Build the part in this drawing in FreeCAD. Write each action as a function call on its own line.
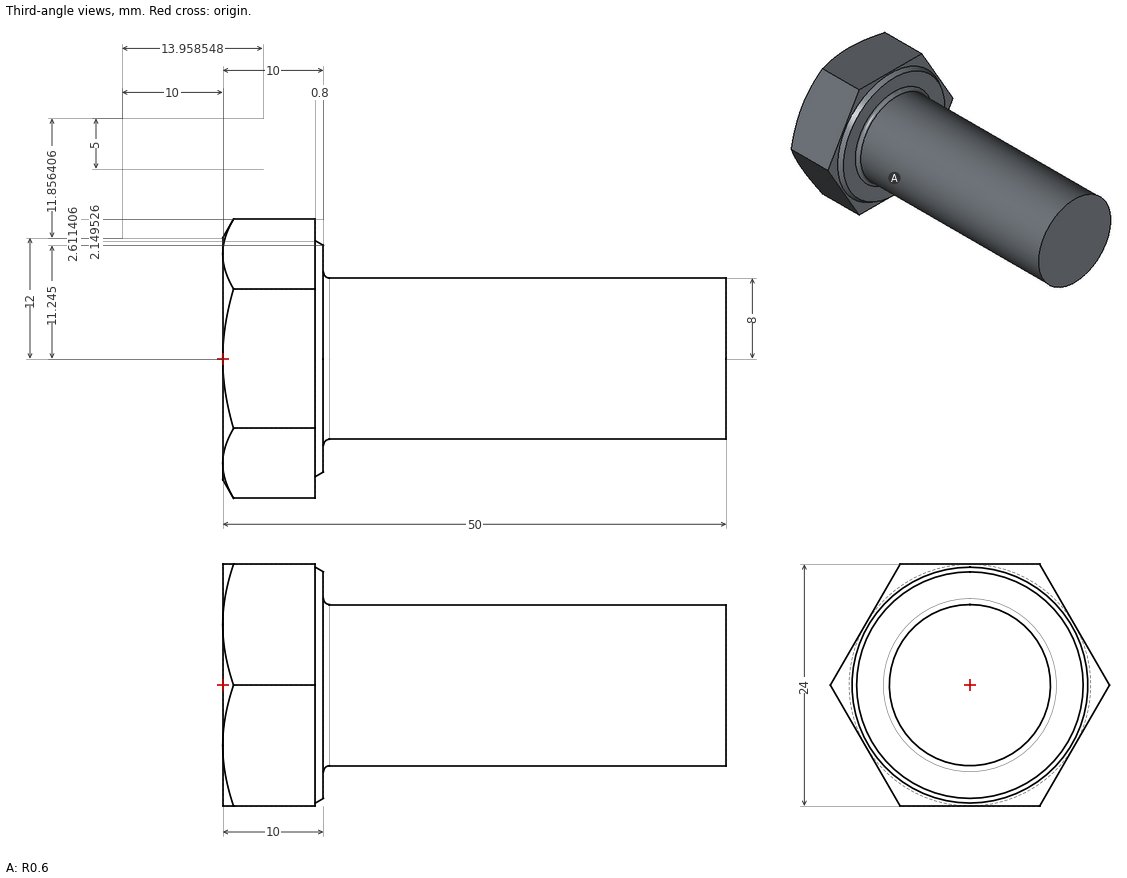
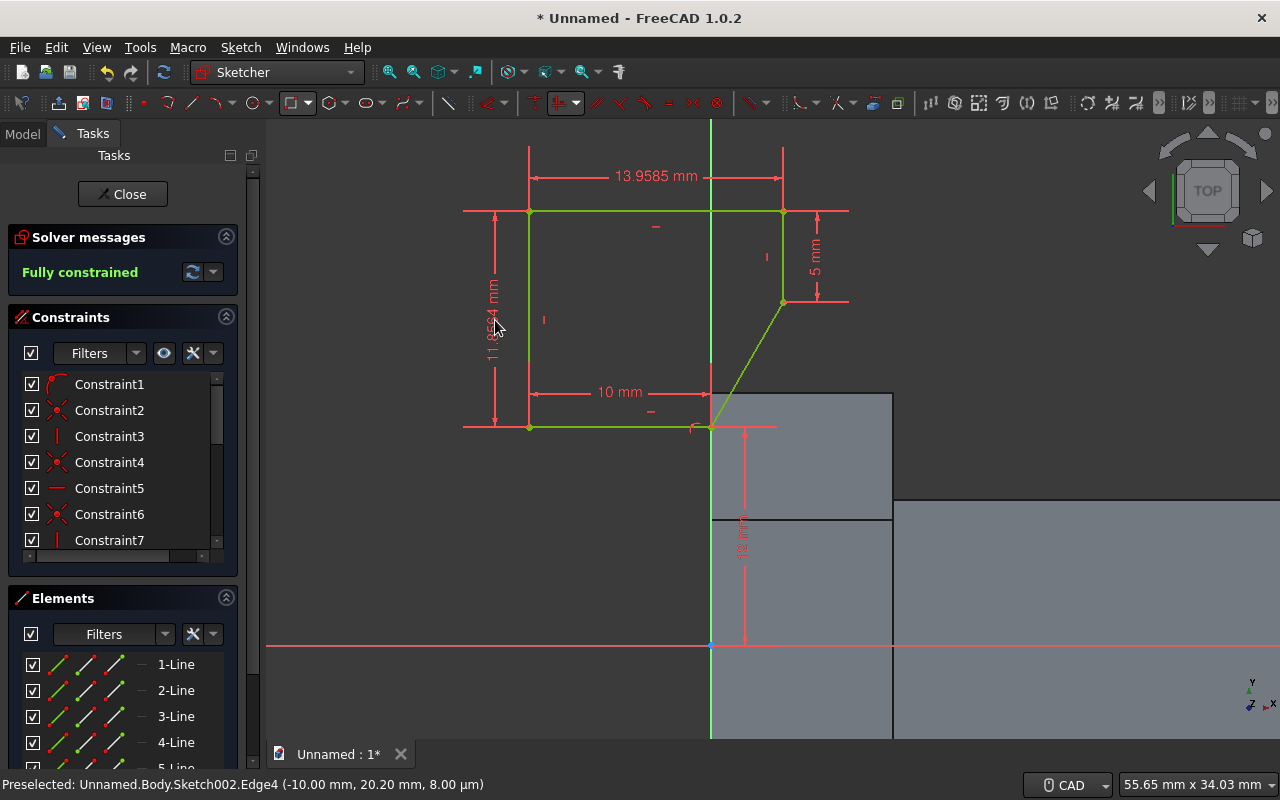
click(123, 194)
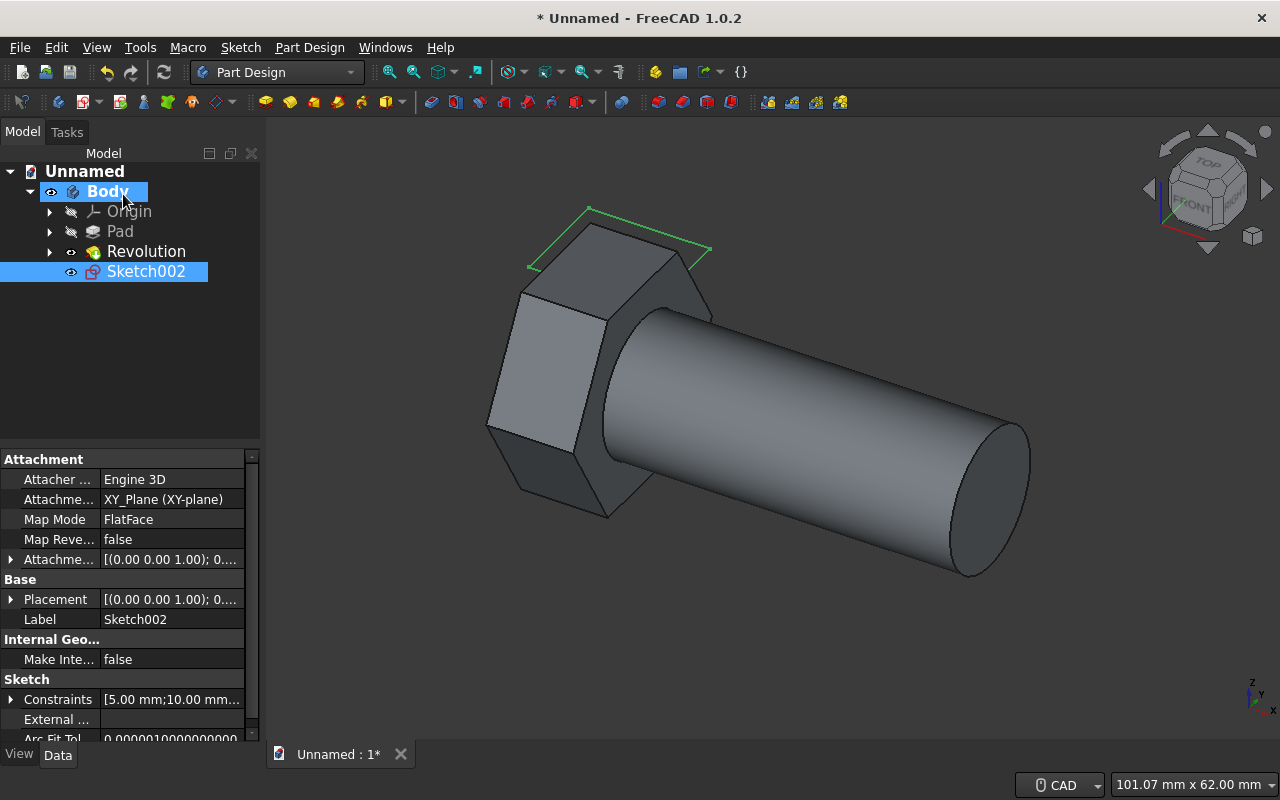
click(480, 102)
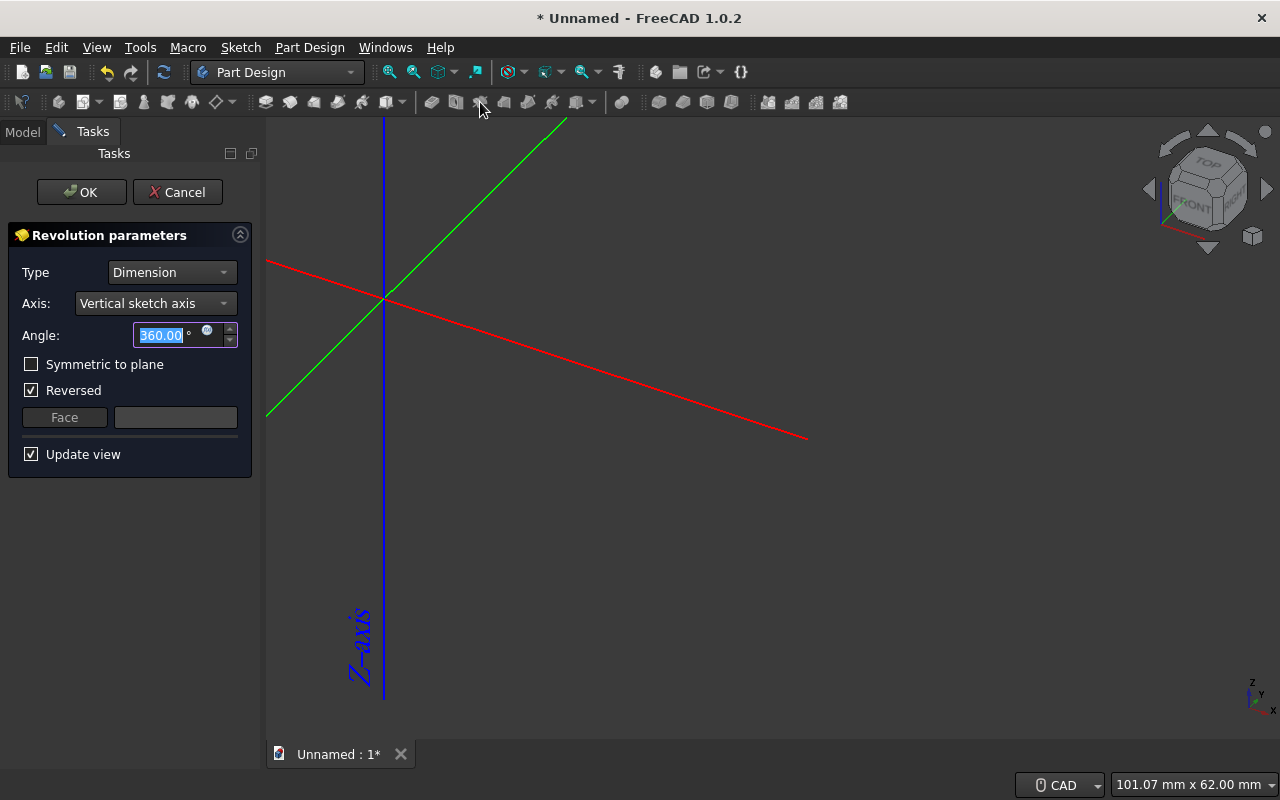
click(156, 304)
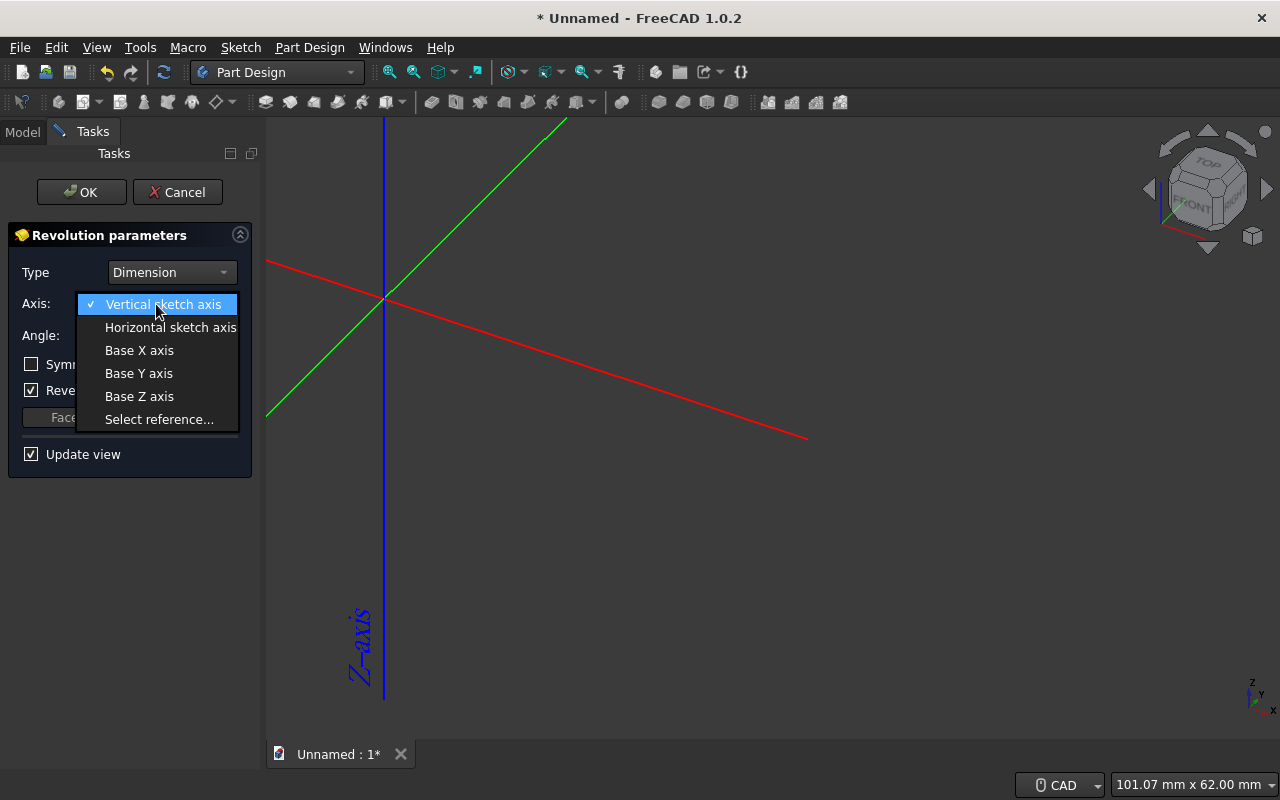
click(156, 328)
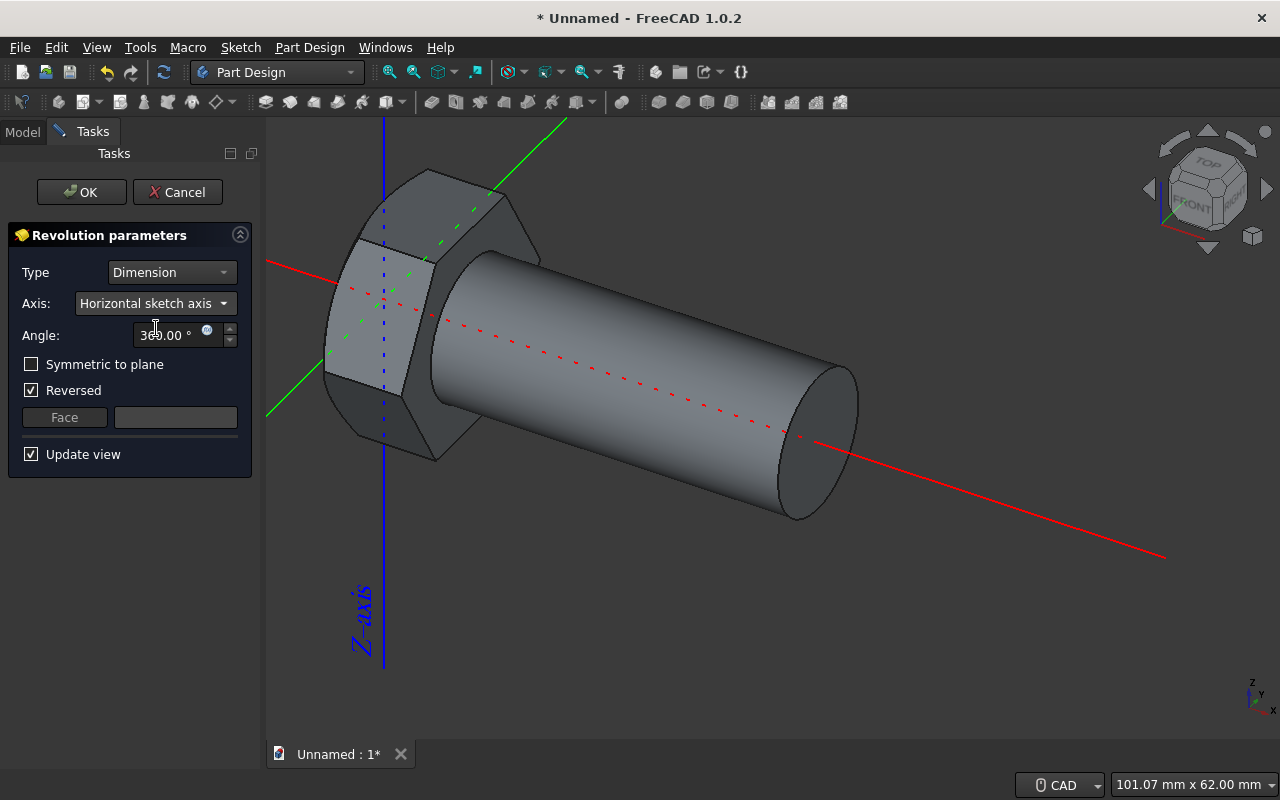
click(82, 192)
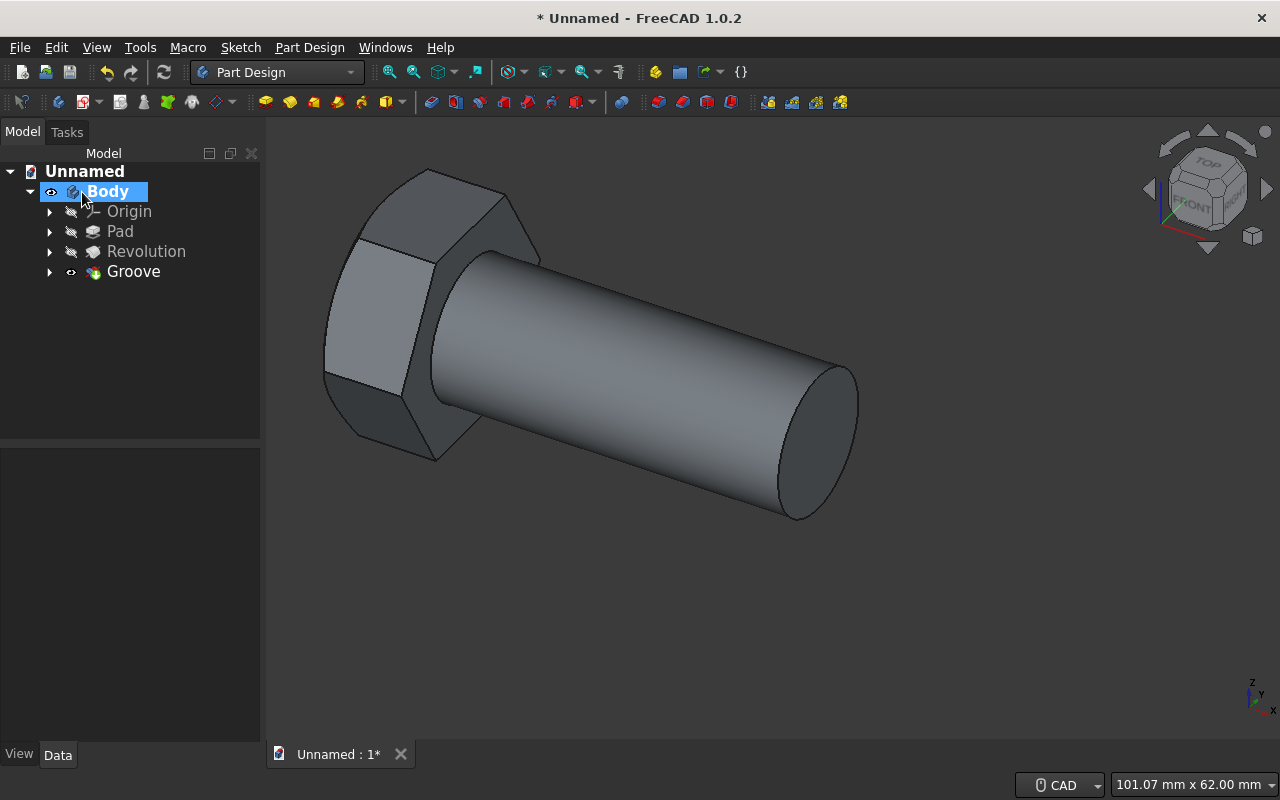
click(84, 102)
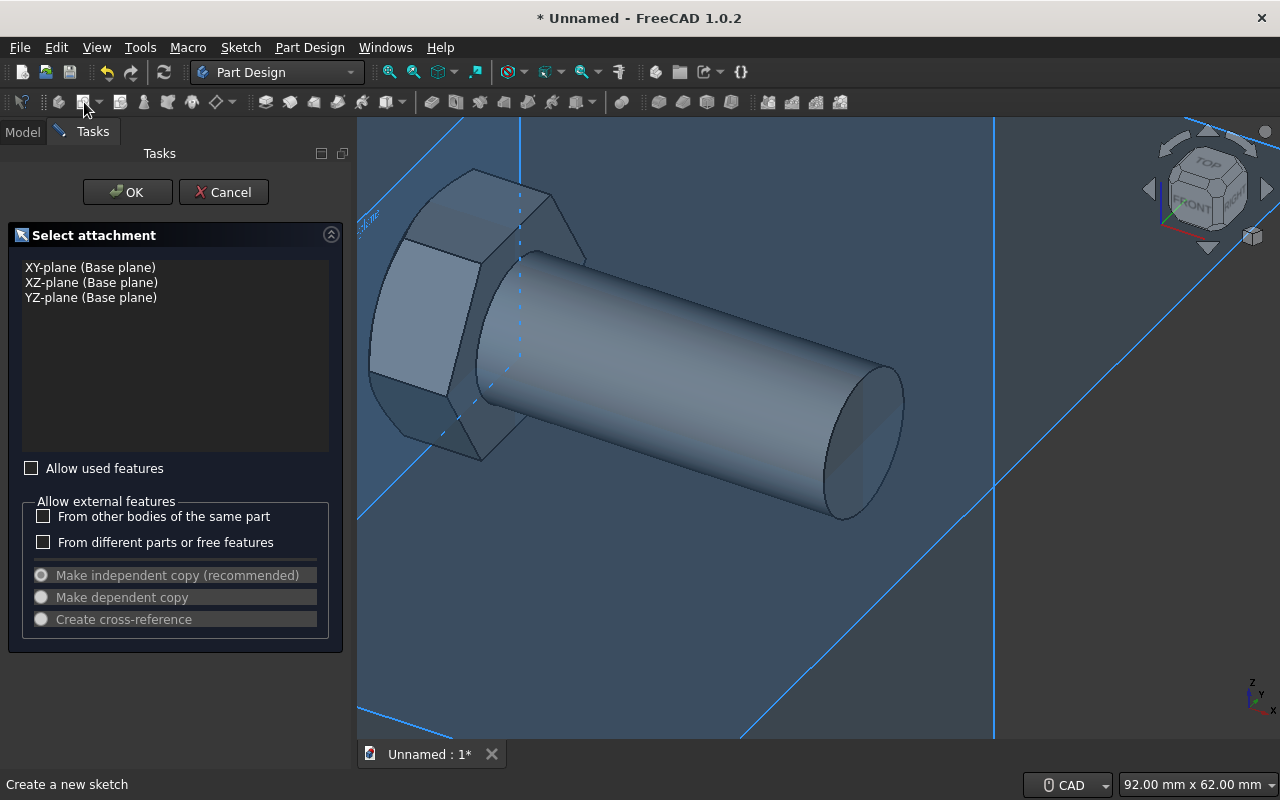
click(82, 268)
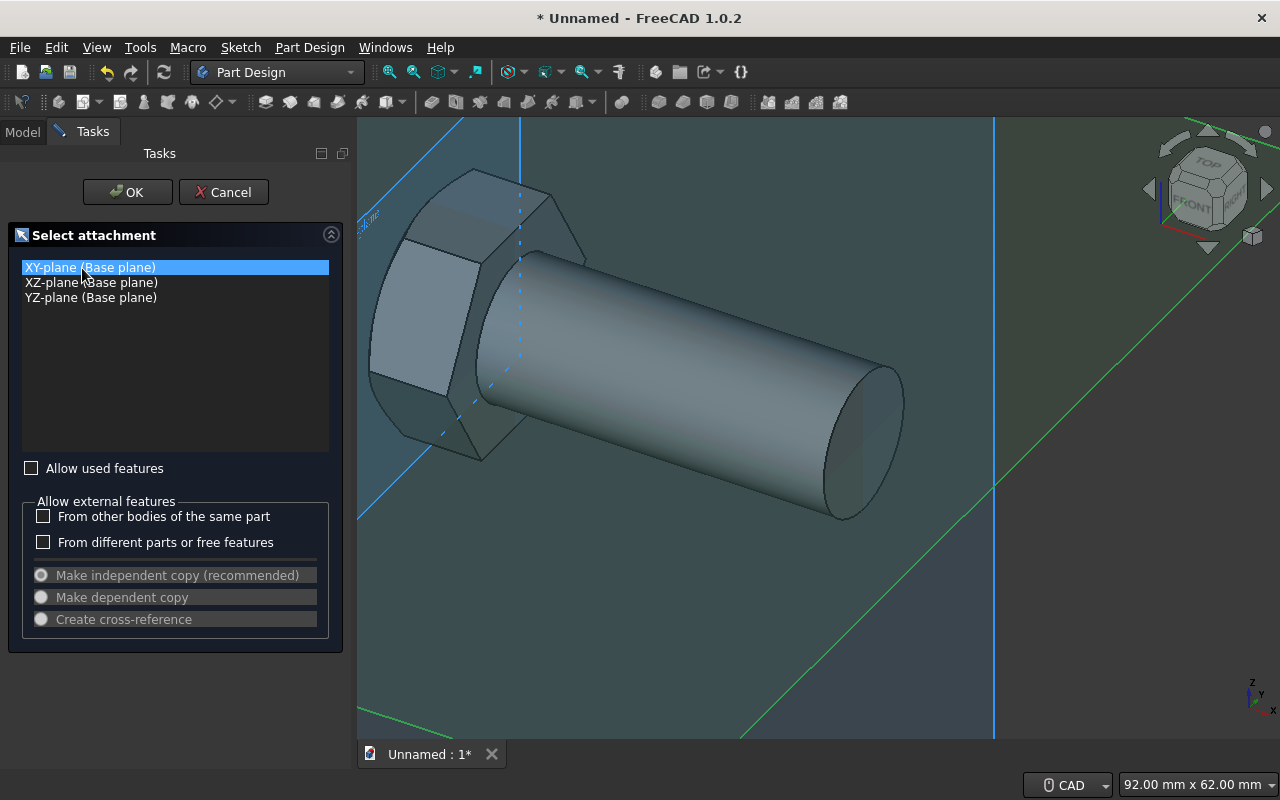
click(128, 192)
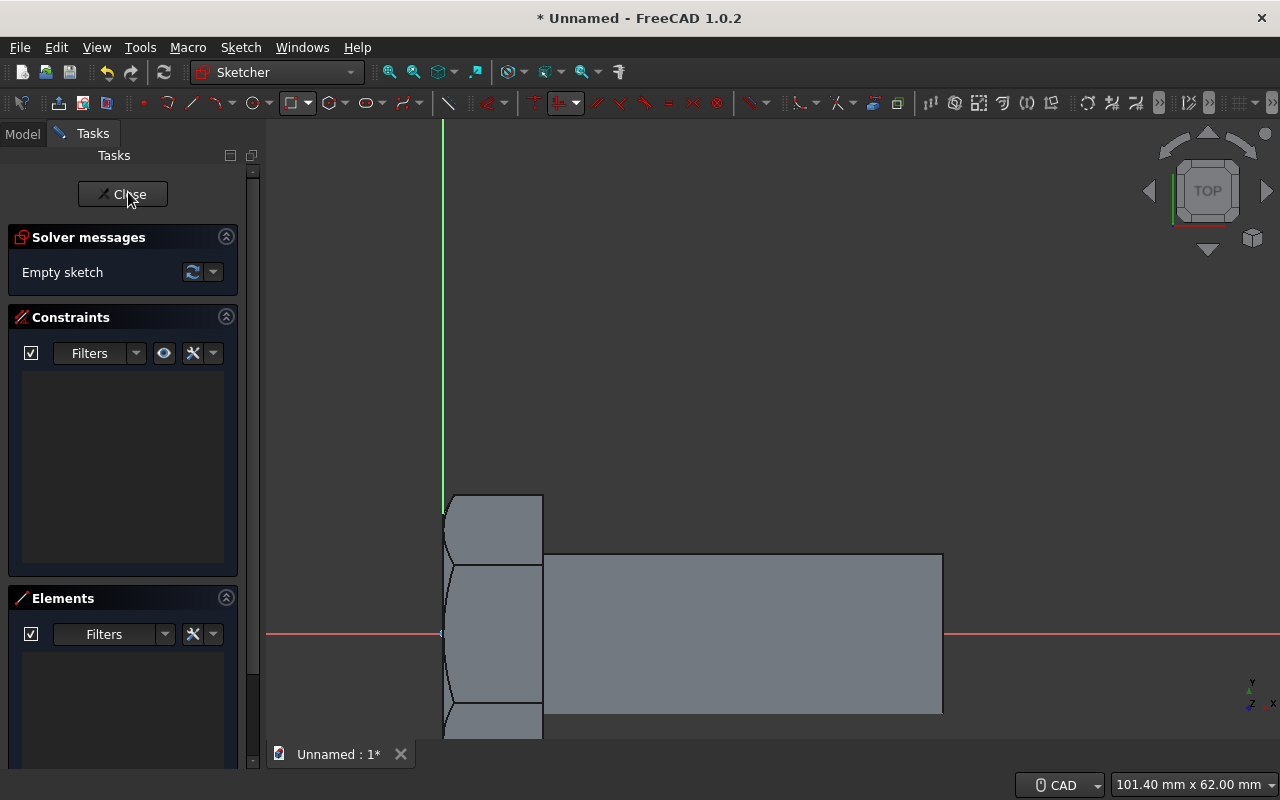
click(108, 104)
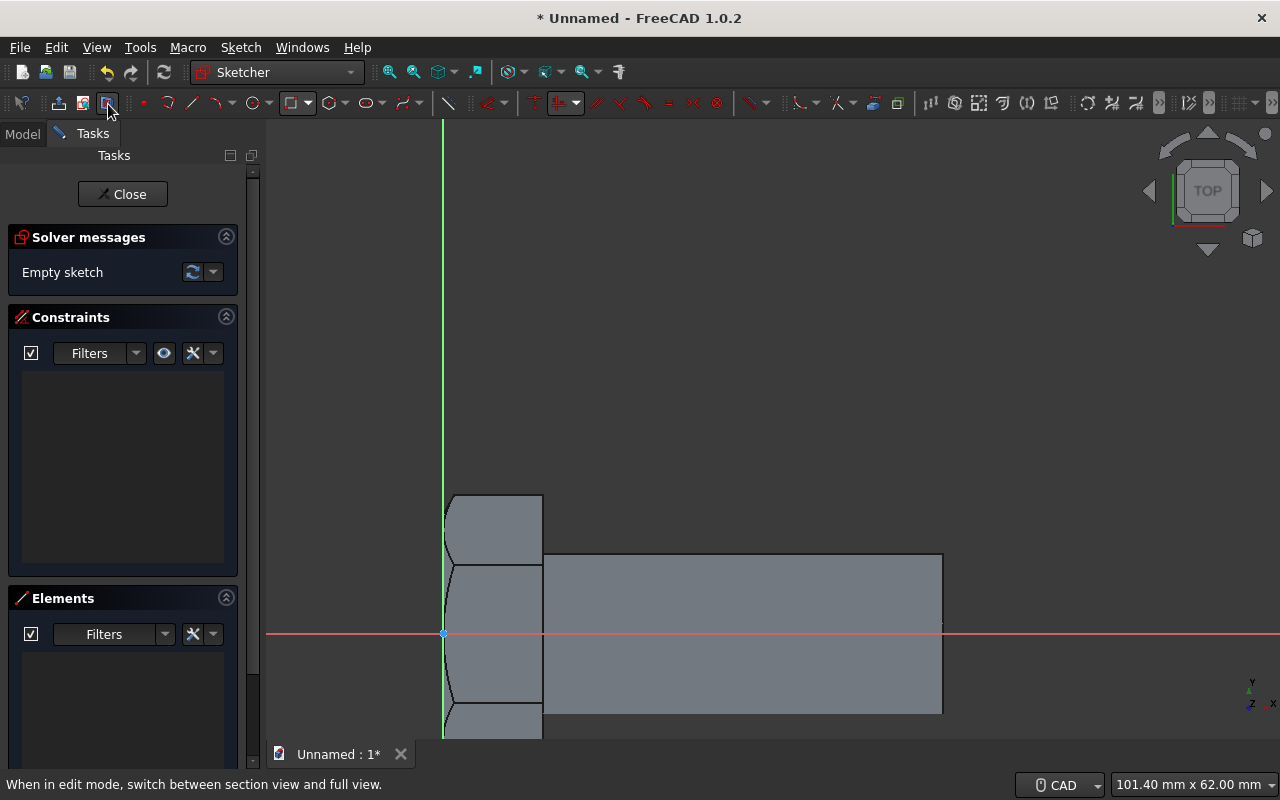
scroll(529, 514, up, 14)